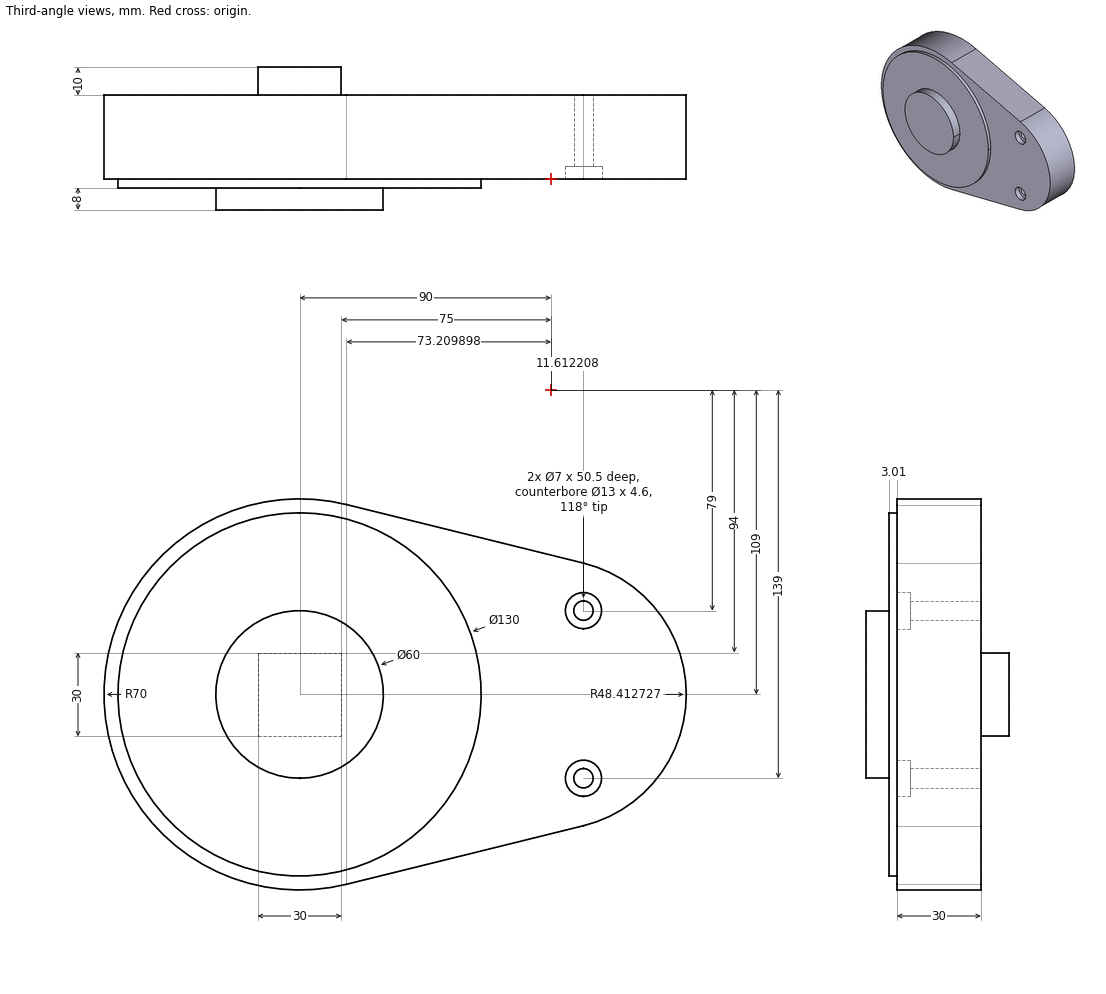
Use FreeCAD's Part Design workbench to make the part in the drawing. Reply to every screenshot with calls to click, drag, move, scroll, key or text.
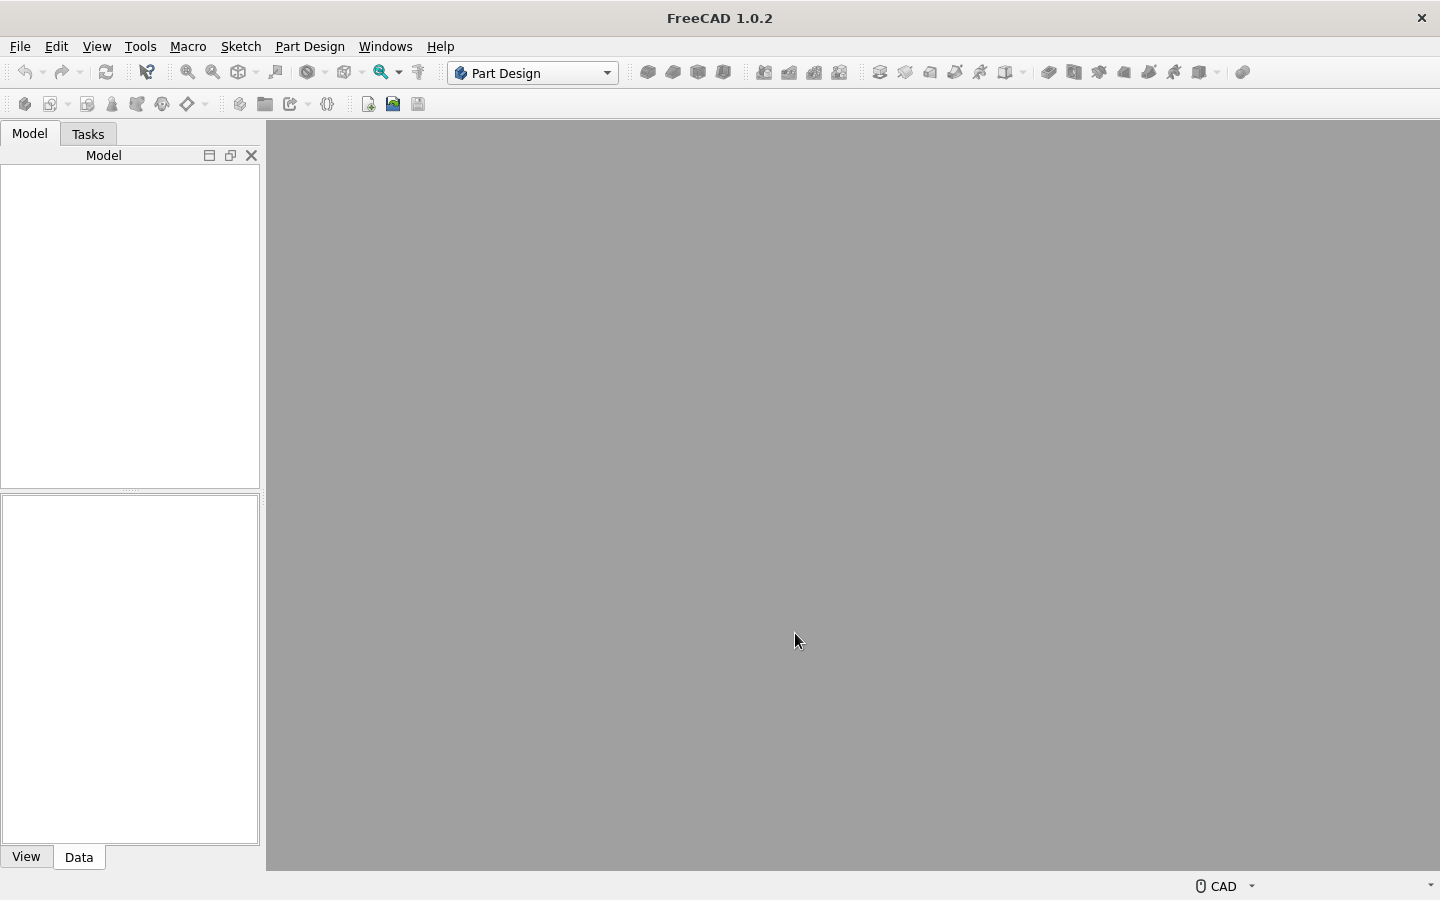
key(ctrl+n)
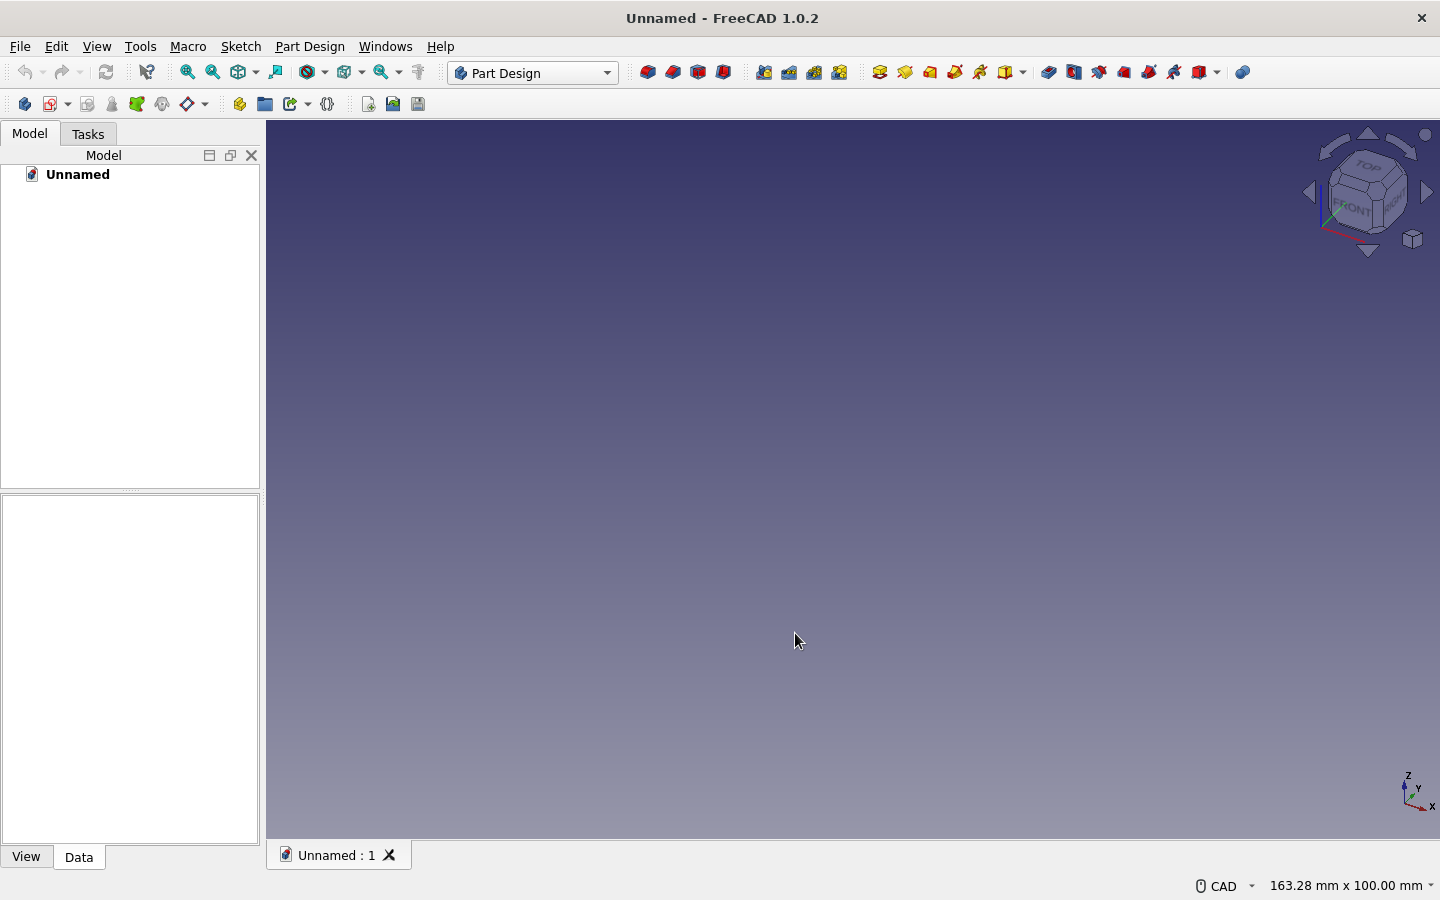
click(50, 104)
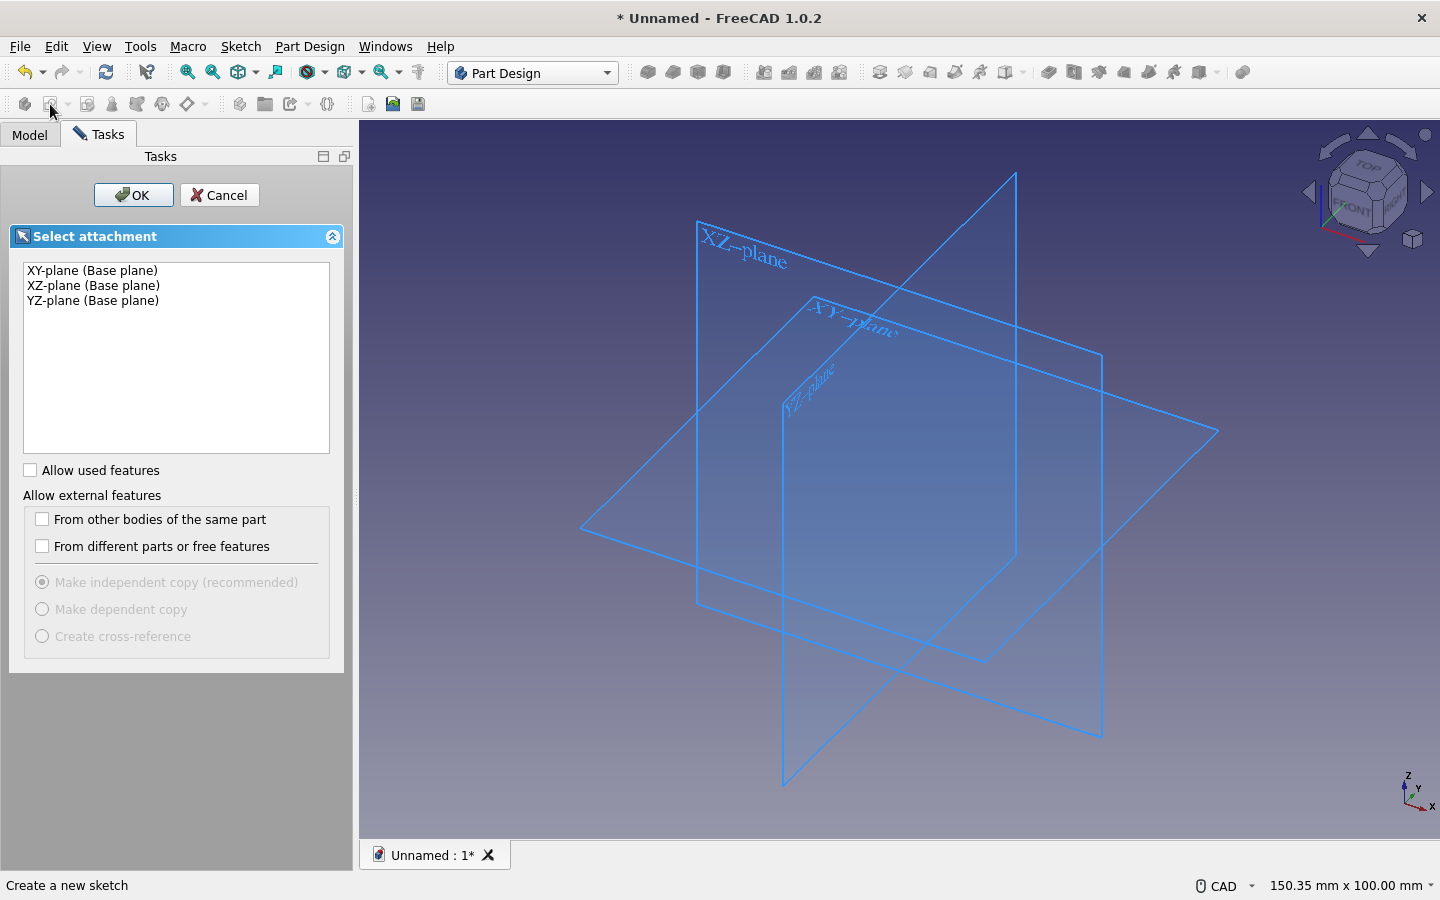
click(84, 286)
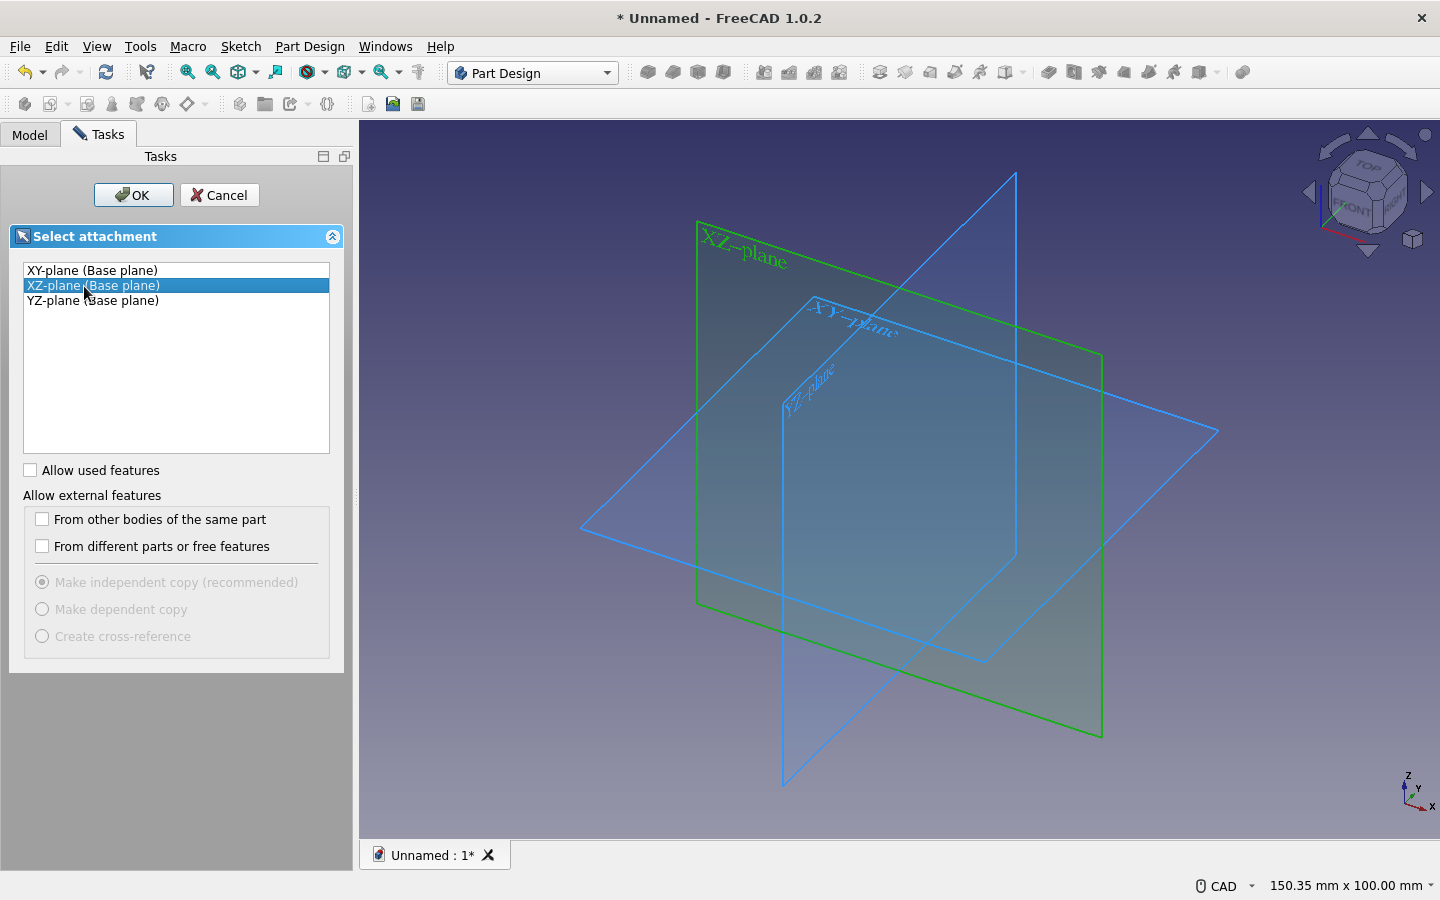
click(134, 195)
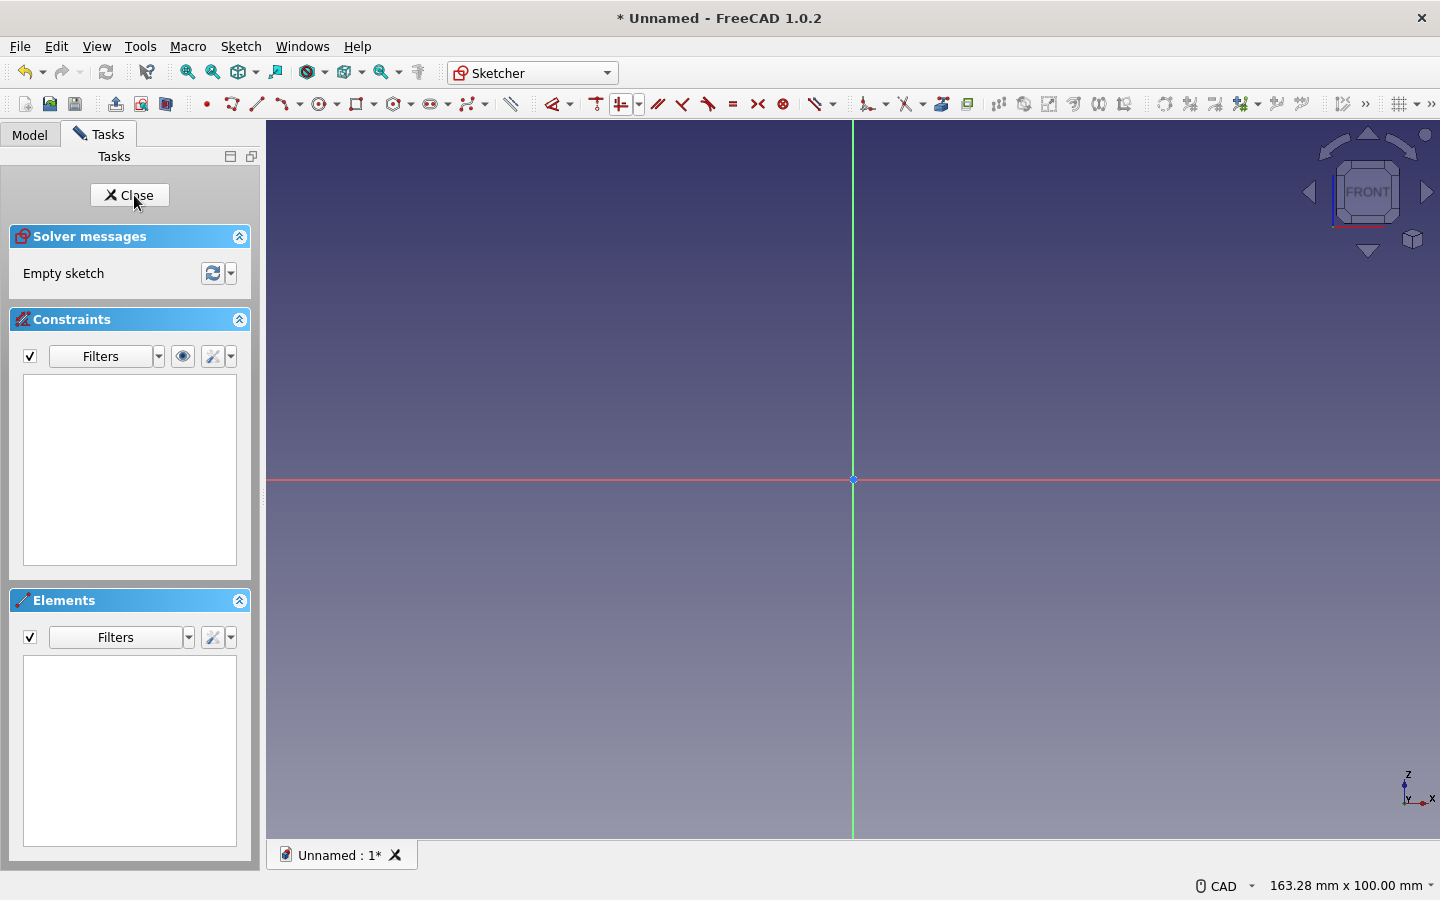
scroll(978, 148, down, 5)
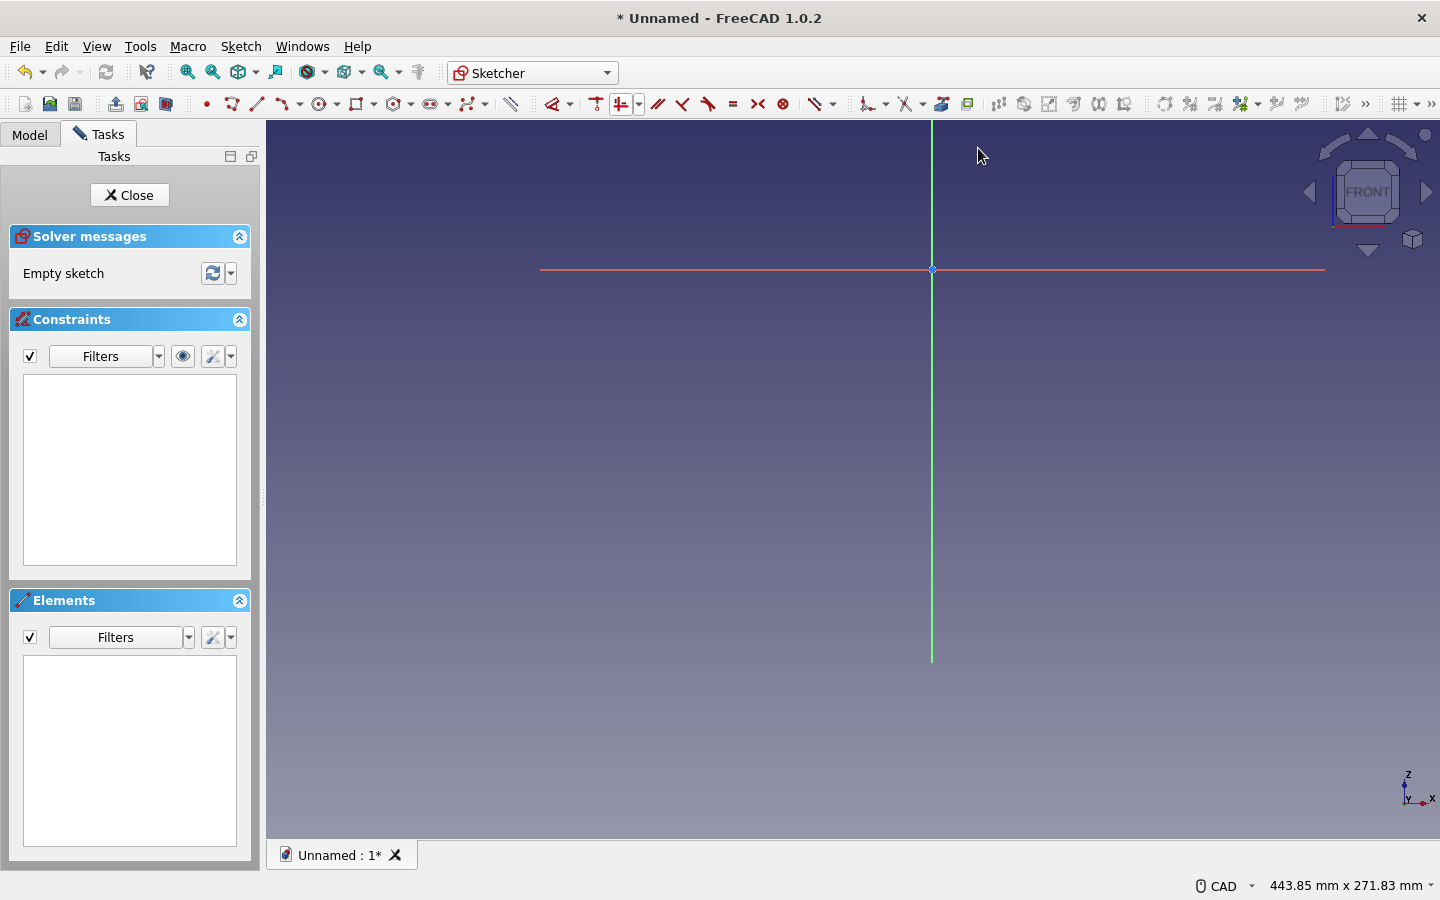
key(g)
key(l)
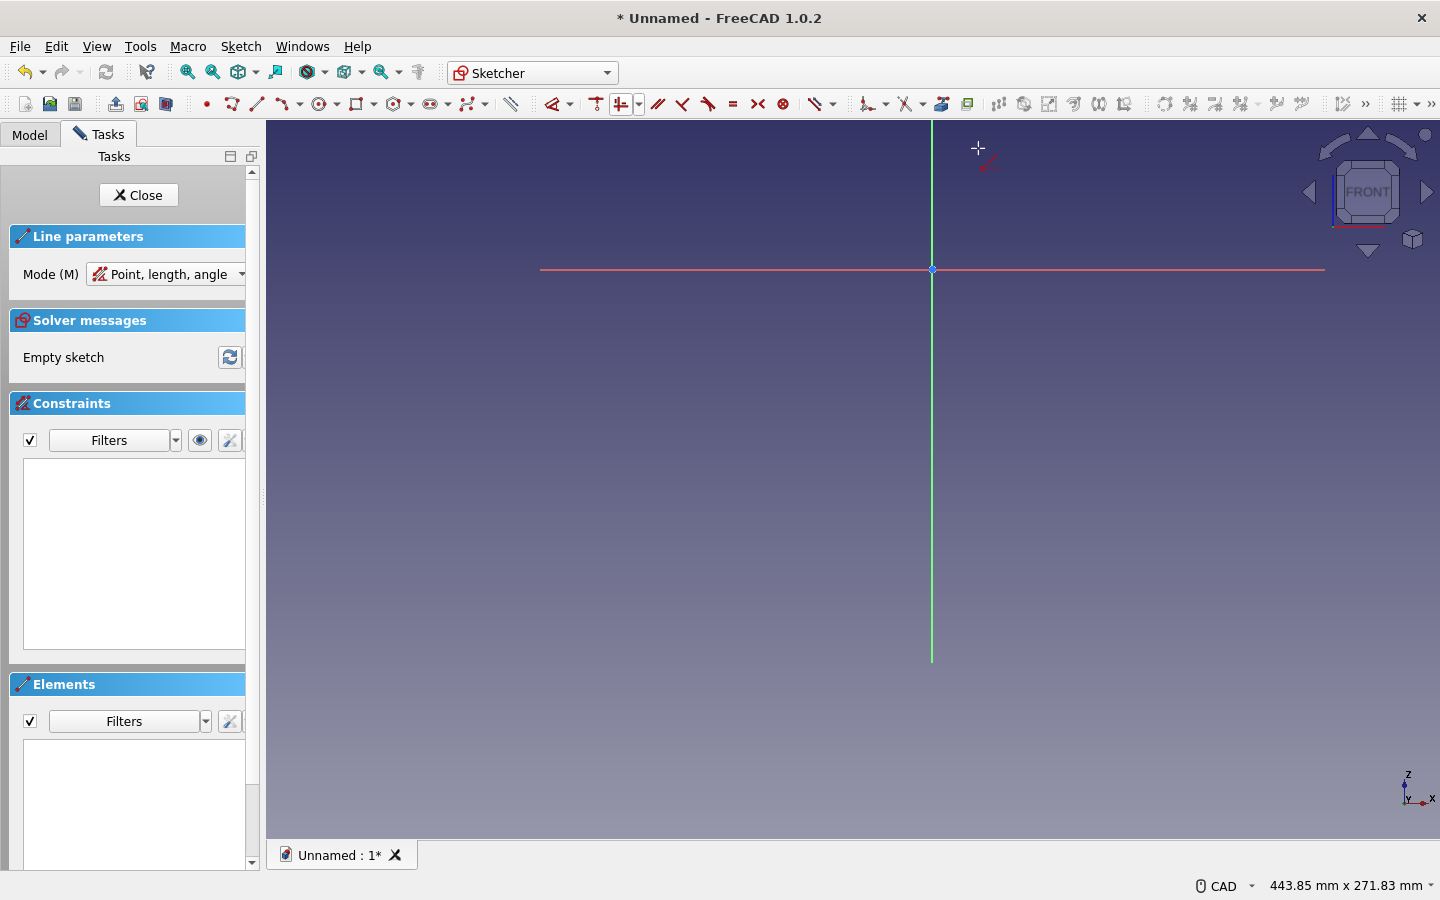
click(963, 683)
click(739, 738)